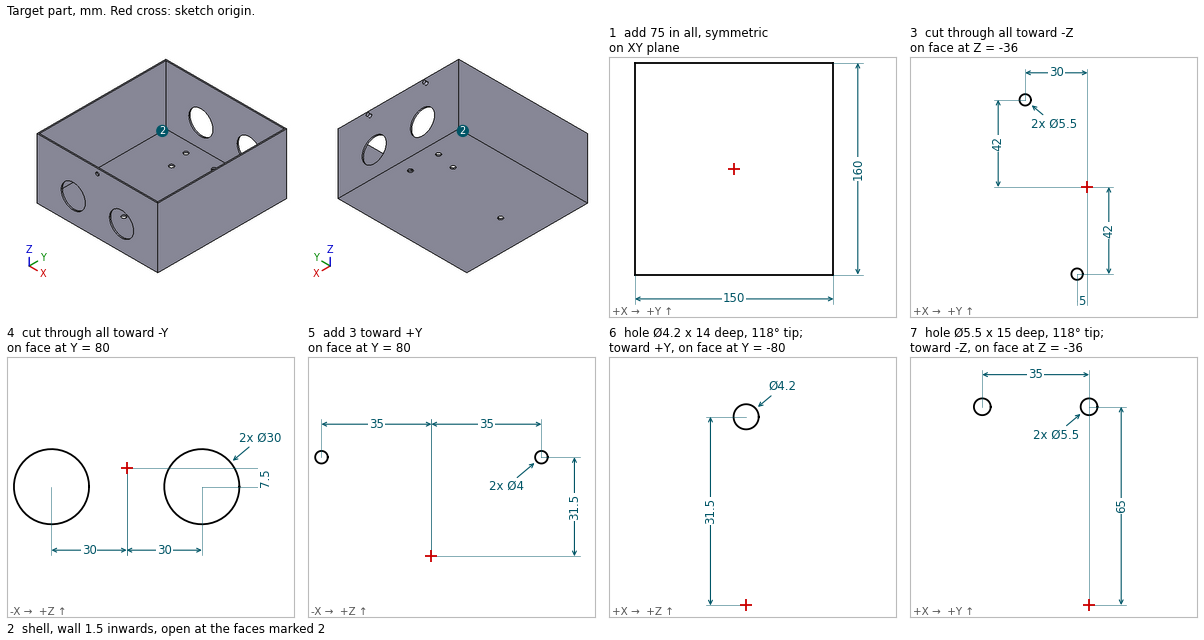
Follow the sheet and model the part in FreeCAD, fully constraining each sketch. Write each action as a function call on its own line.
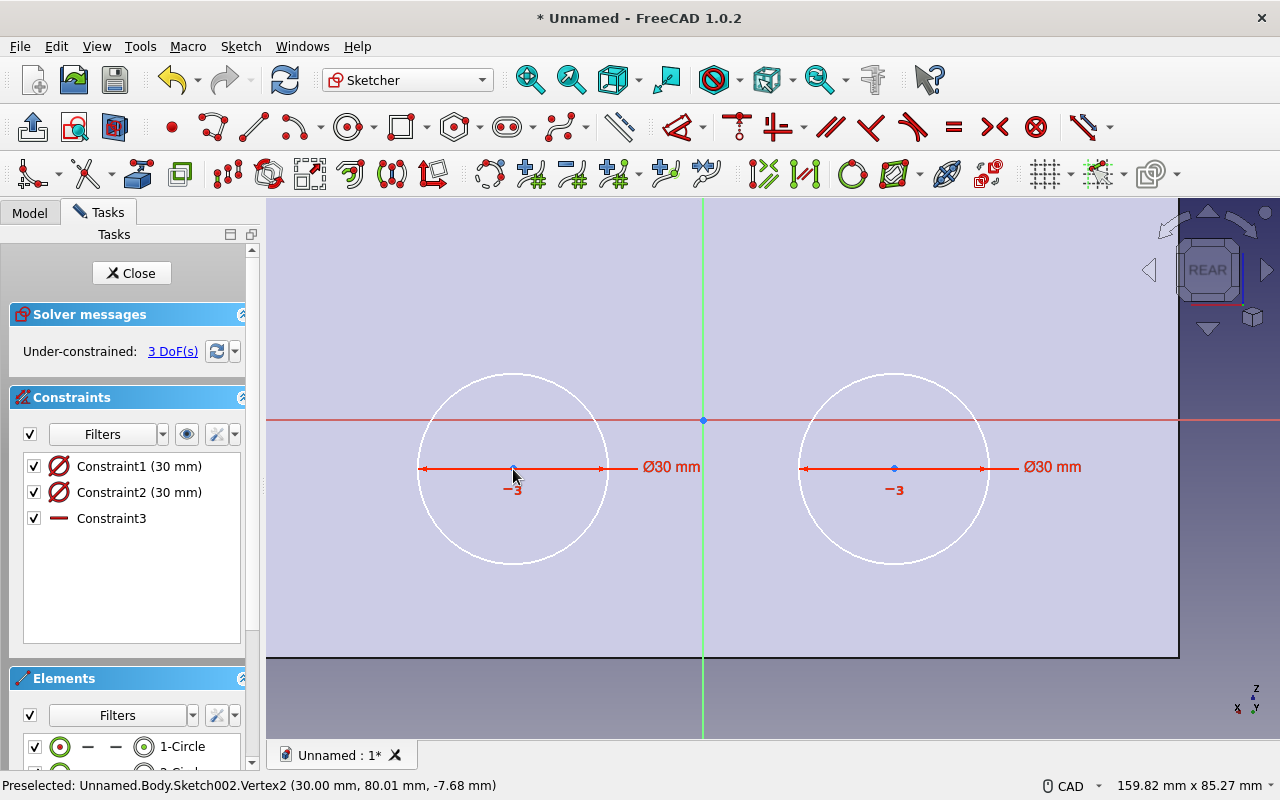
key(d)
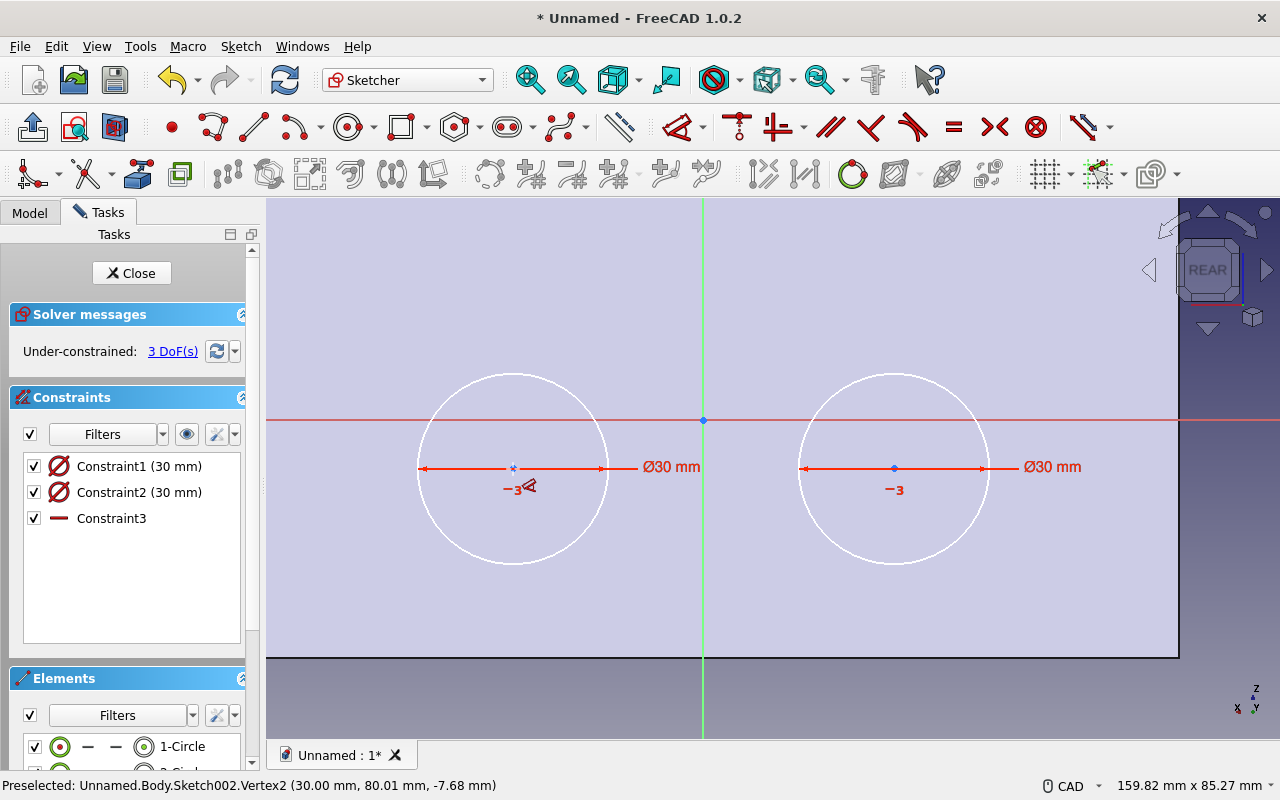
click(894, 469)
click(799, 386)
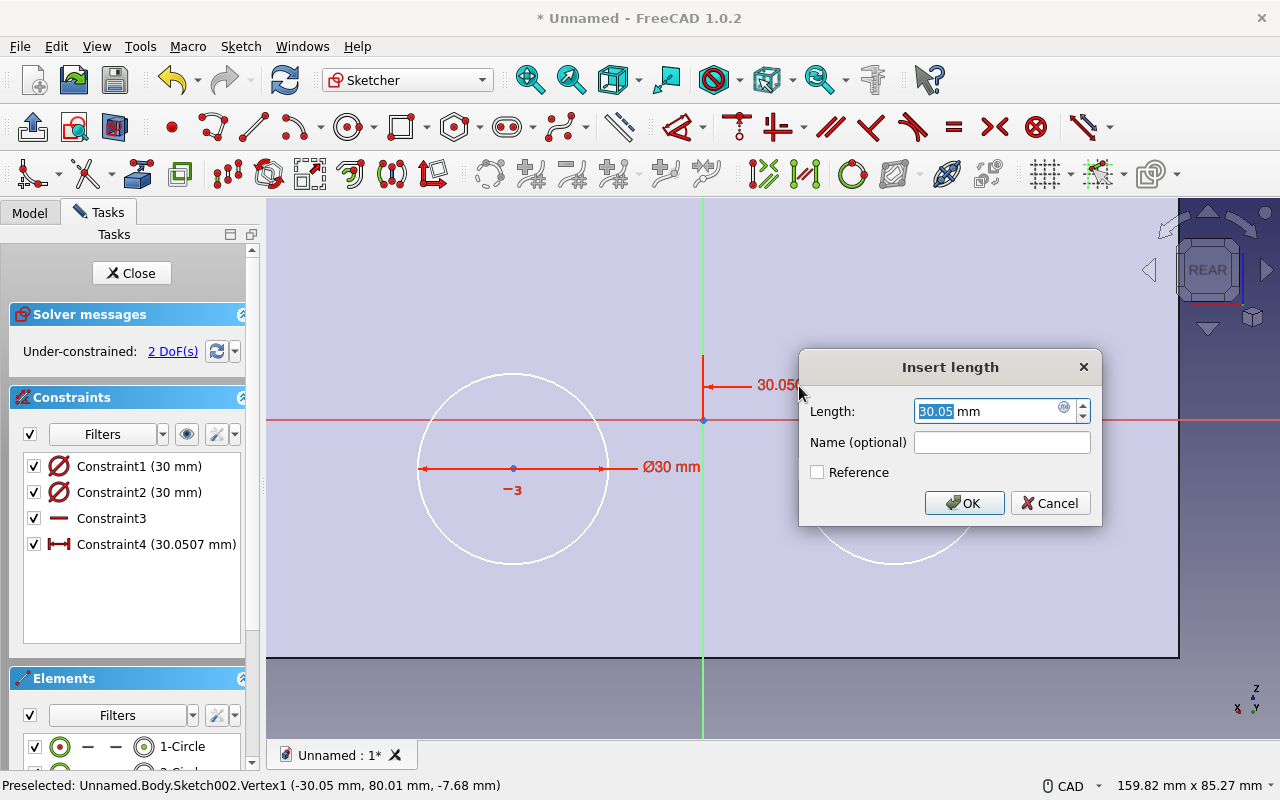
text(30)
key(Return)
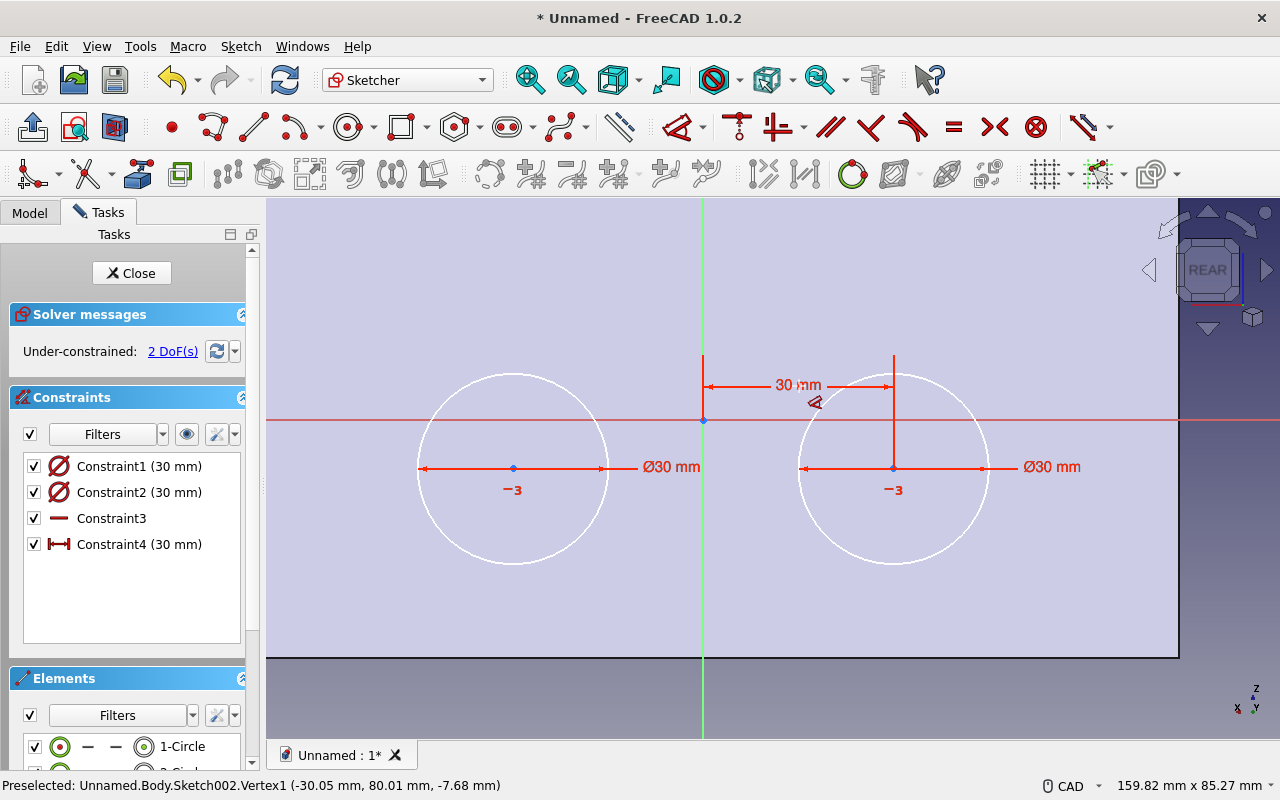
click(513, 469)
click(608, 386)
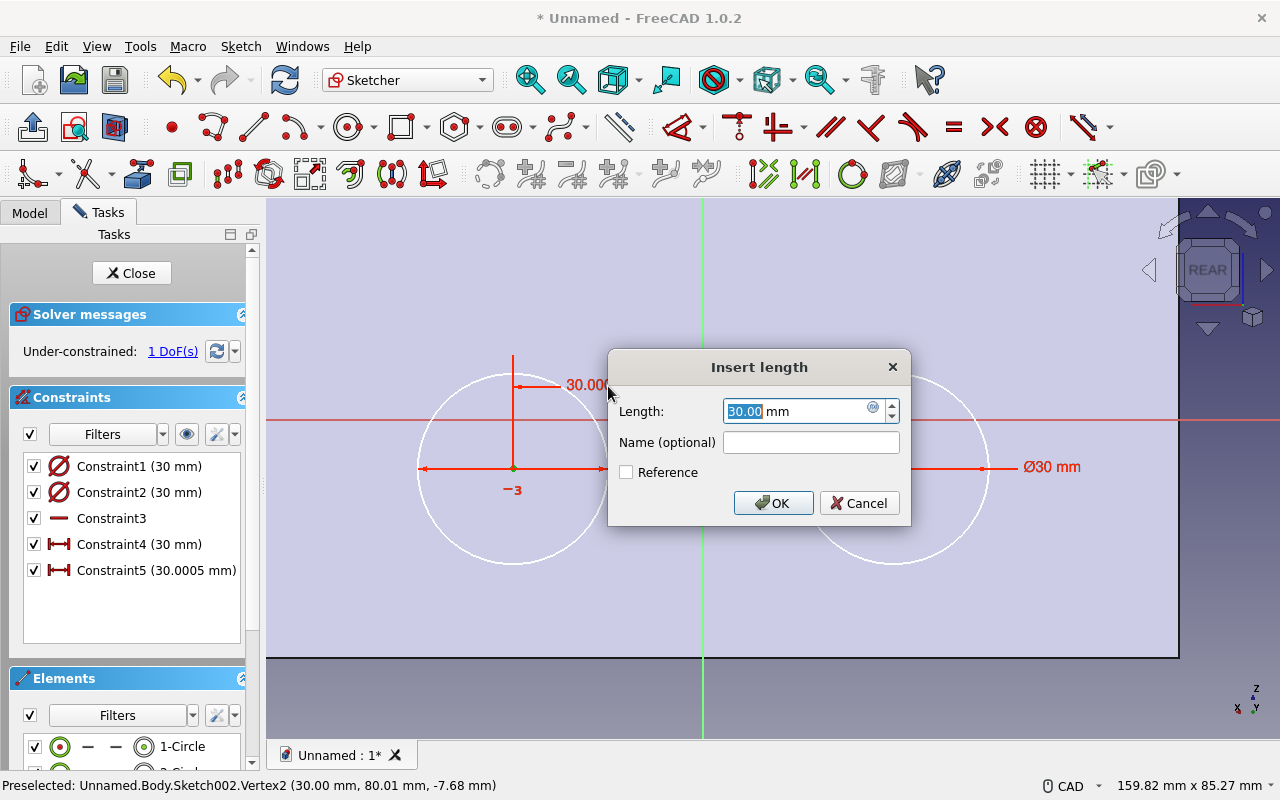
text(30)
key(Return)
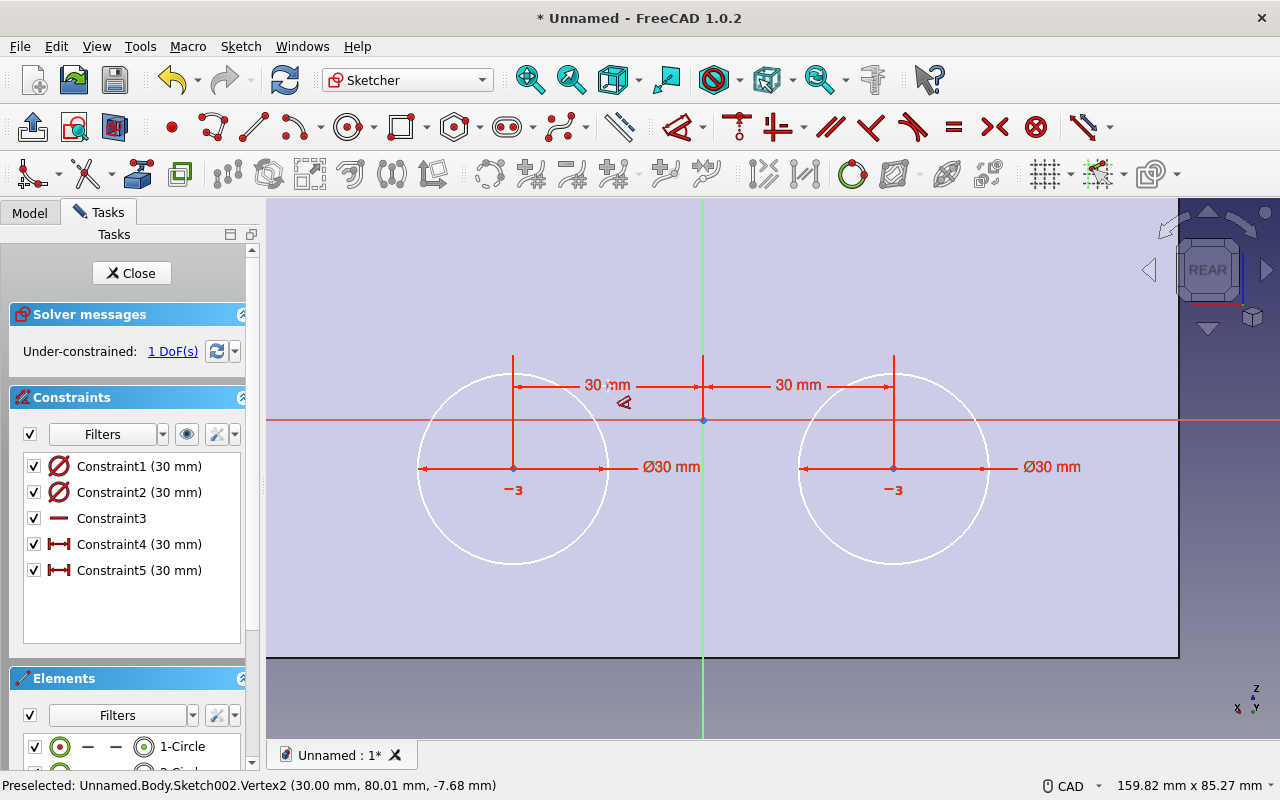
click(894, 469)
click(928, 445)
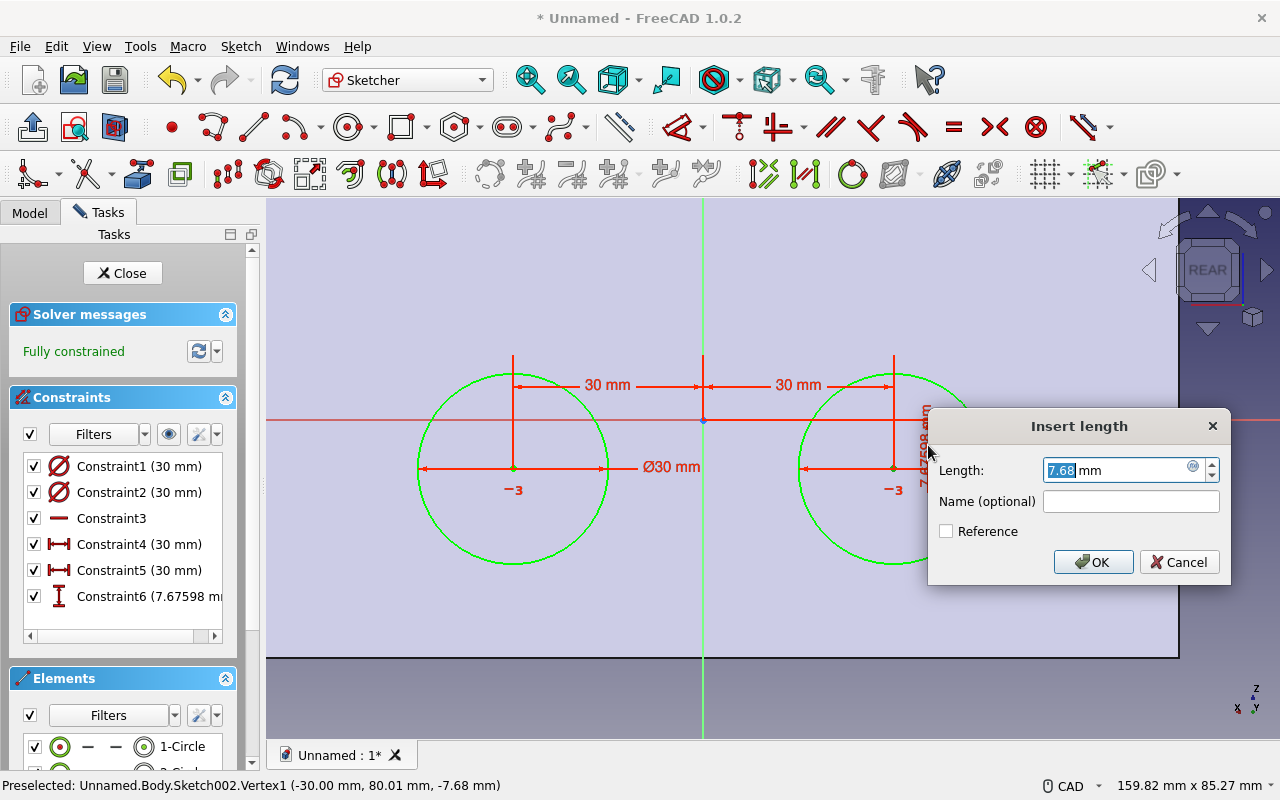
text(7.5)
key(Return)
key(Escape)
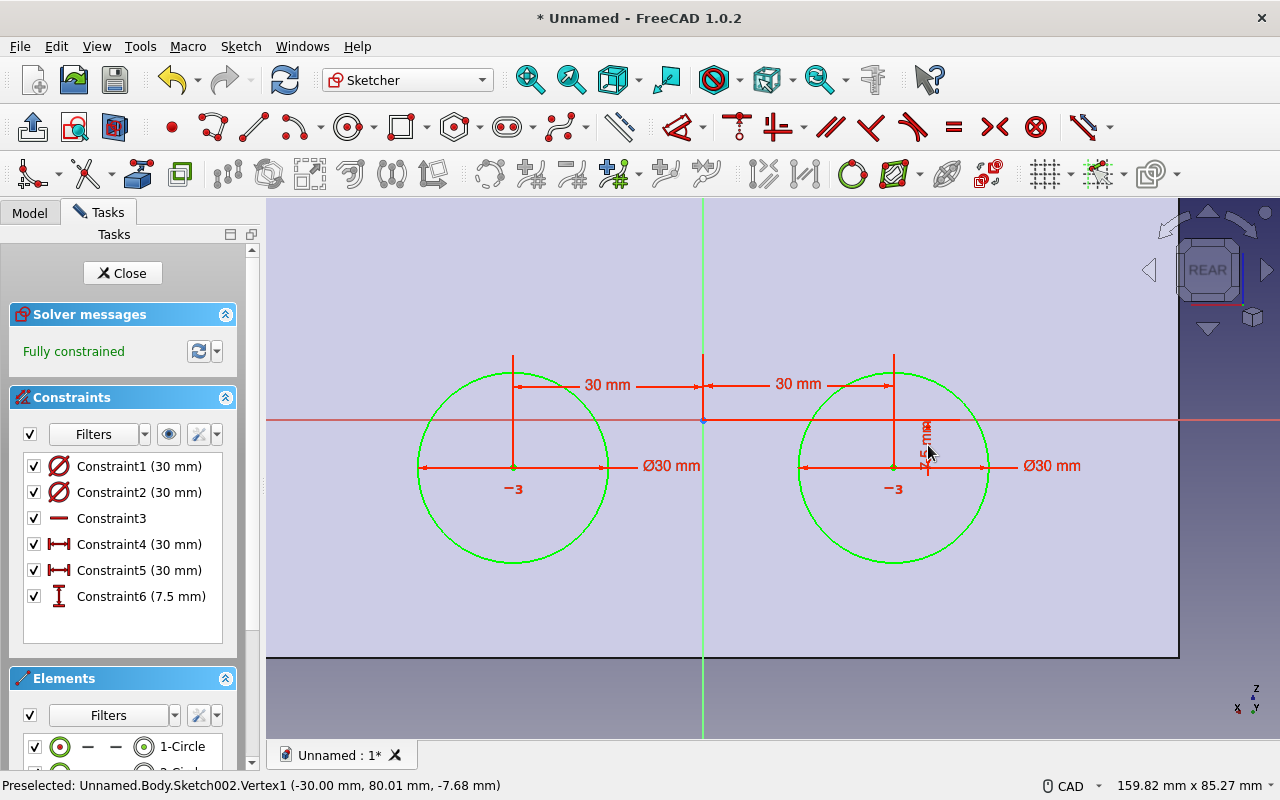
click(123, 273)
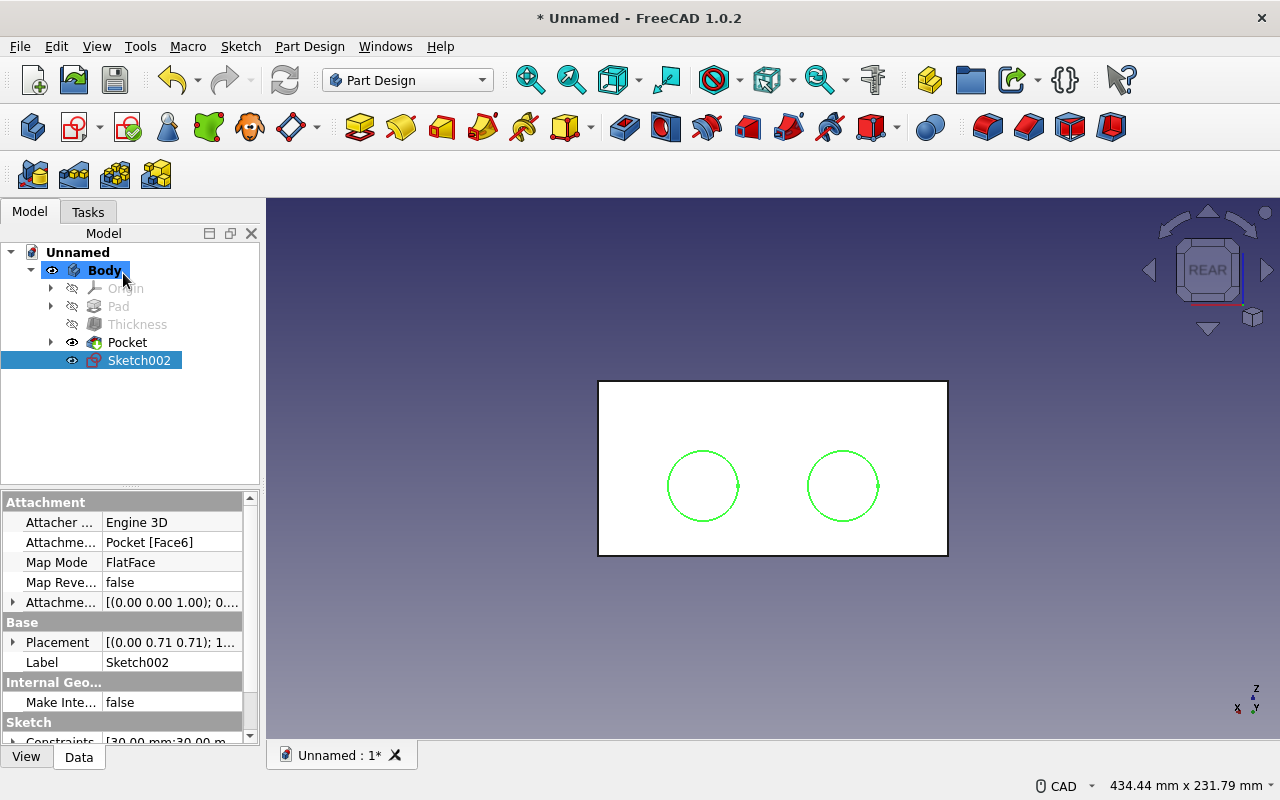
click(625, 128)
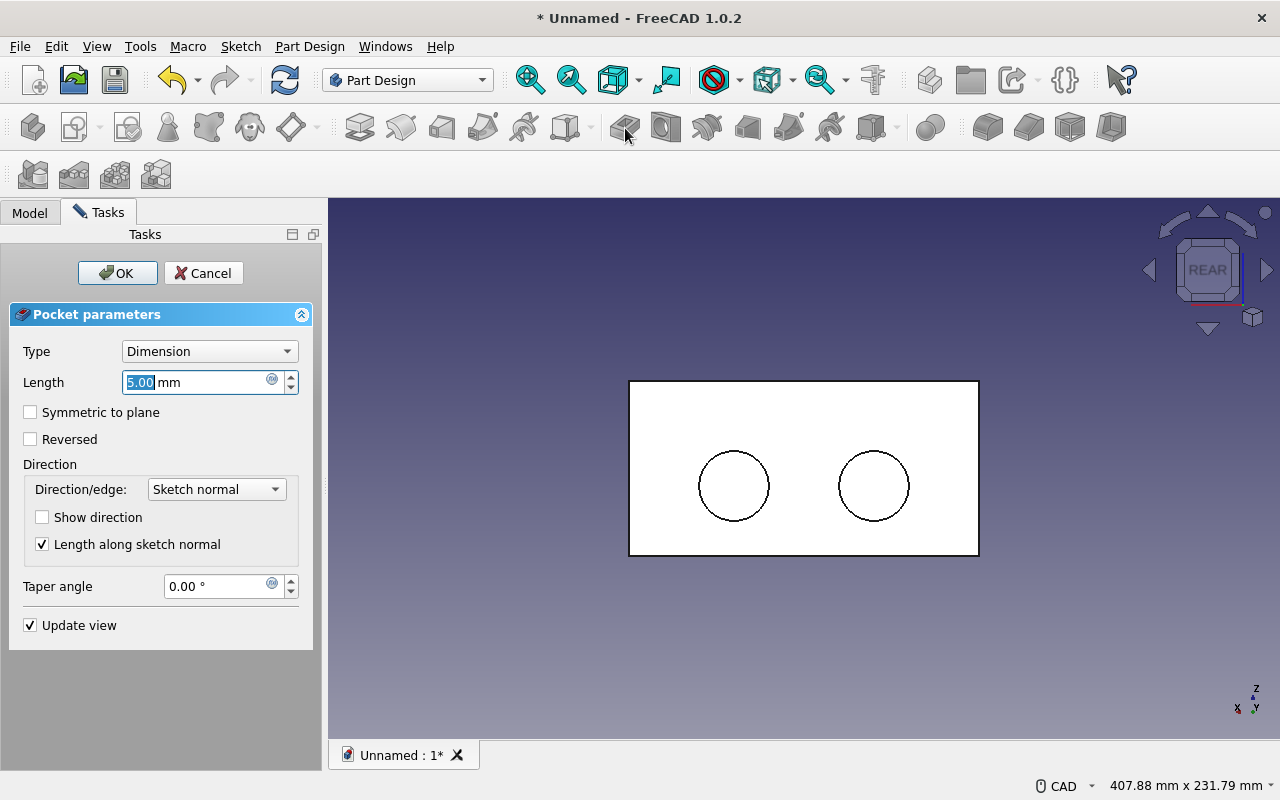
click(210, 352)